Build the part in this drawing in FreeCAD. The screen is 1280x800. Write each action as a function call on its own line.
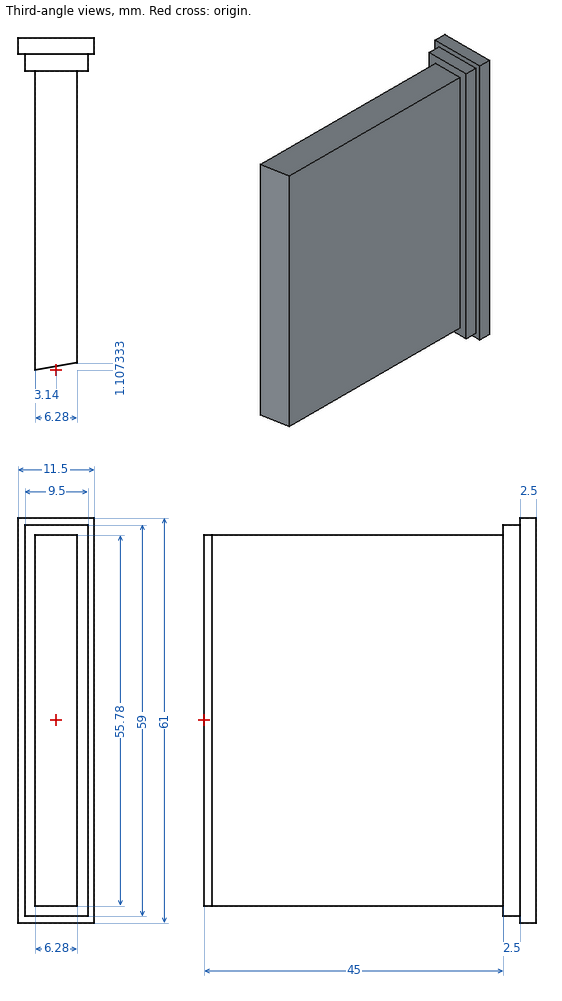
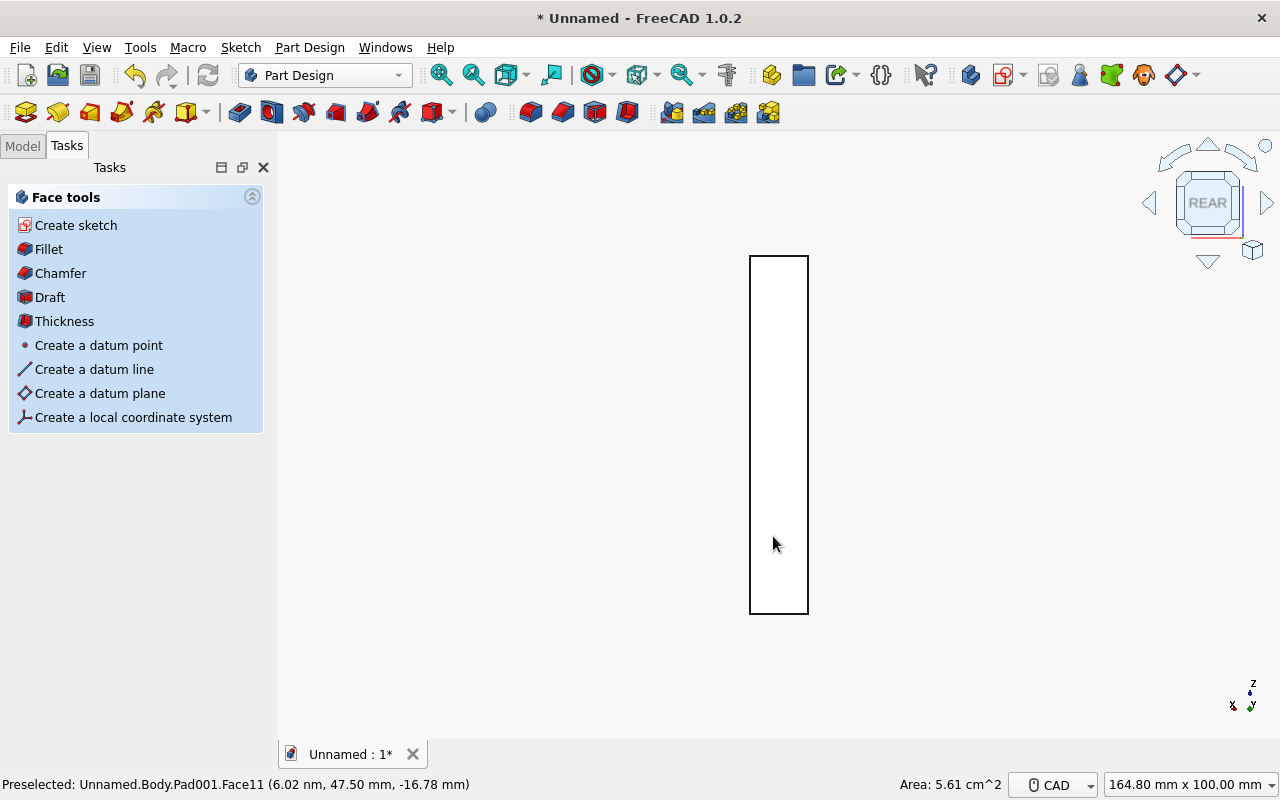
click(1004, 76)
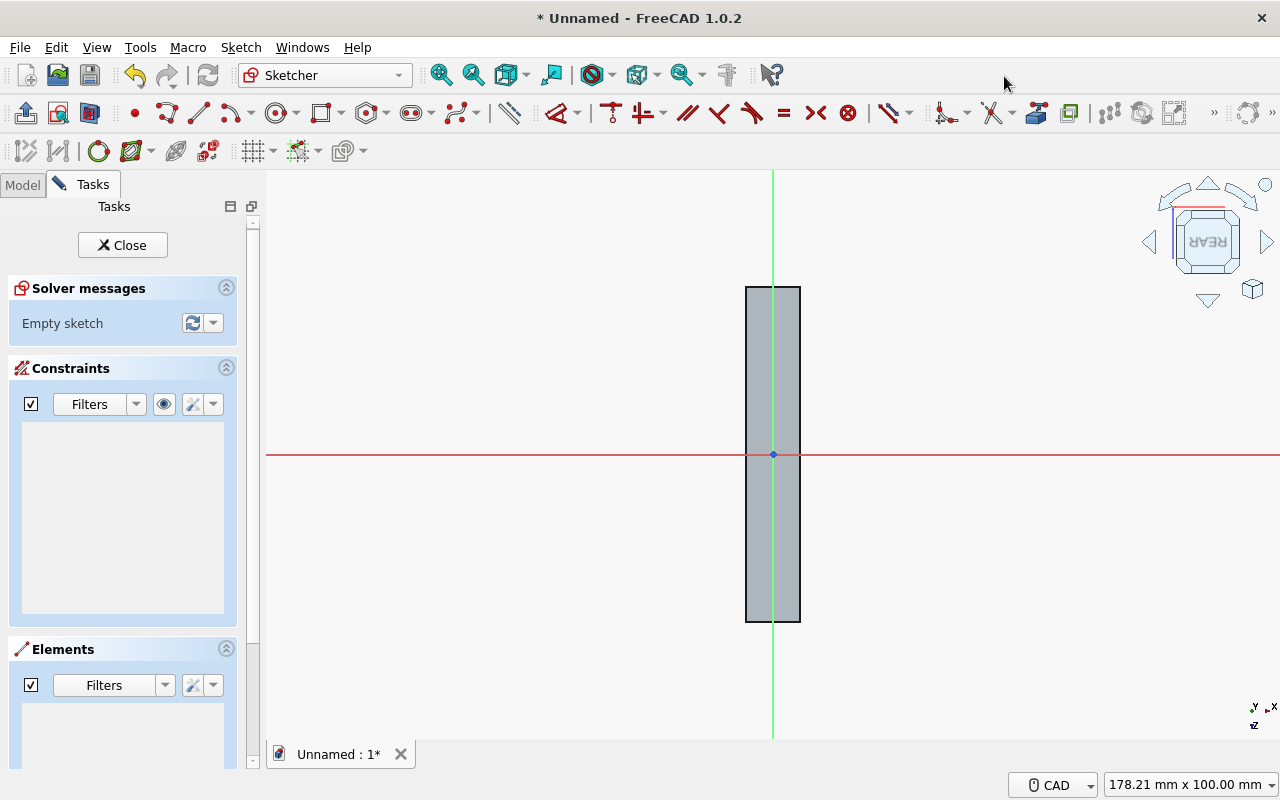
key(g)
key(v)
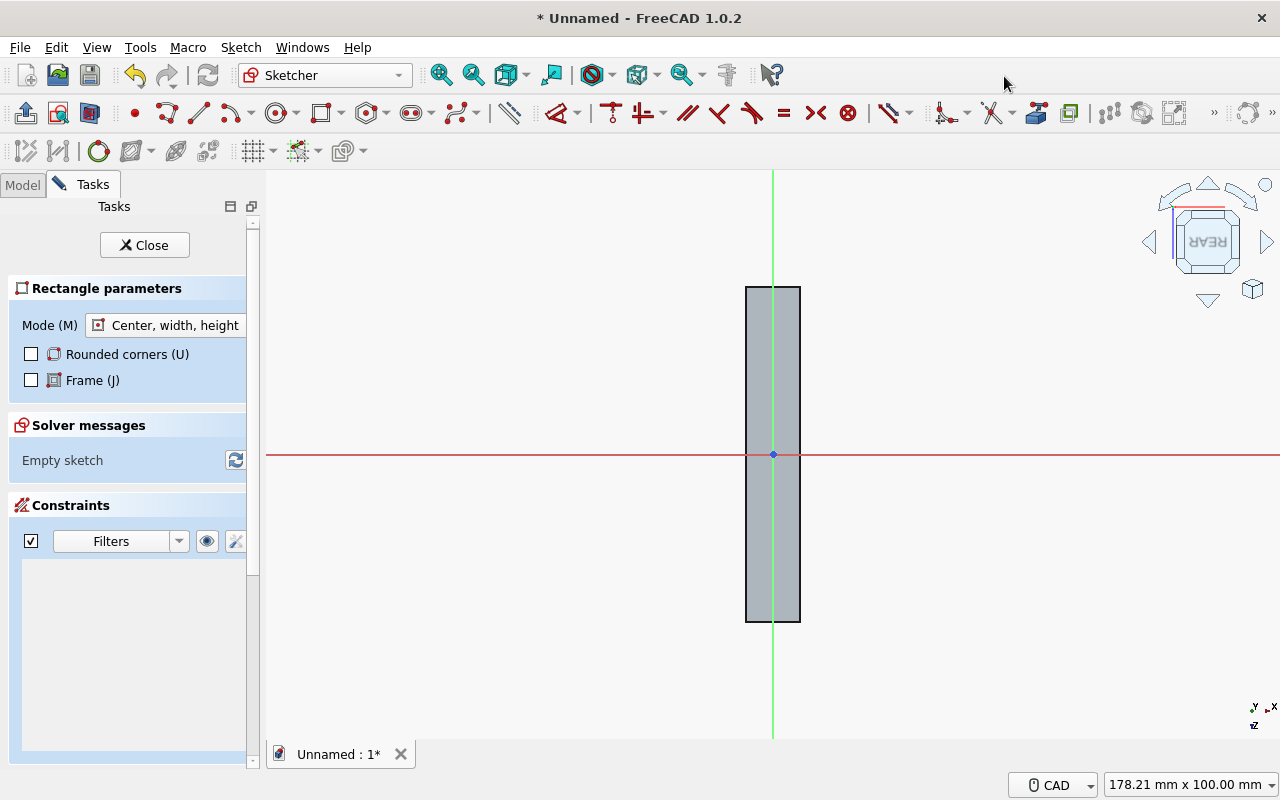
click(773, 454)
move(806, 281)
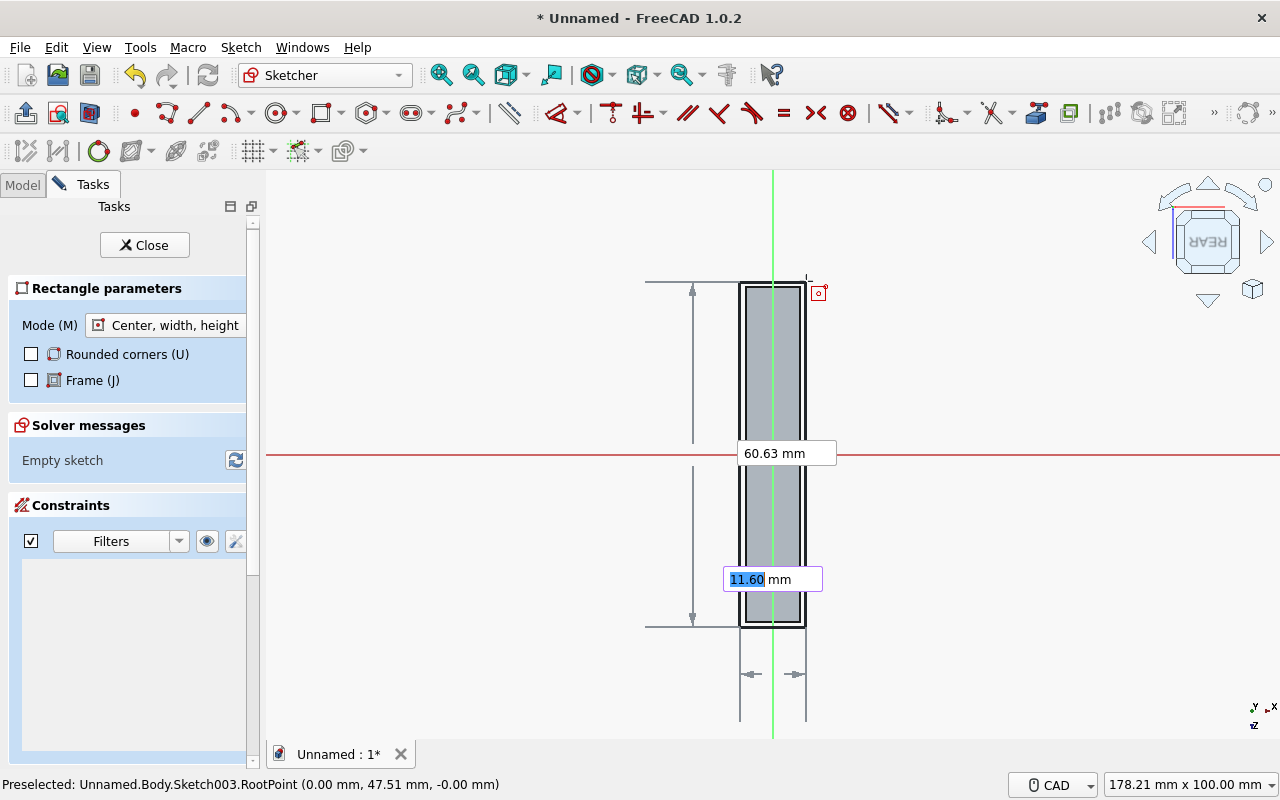
text(11.5)
key(Tab)
text(61)
key(Return)
key(Escape)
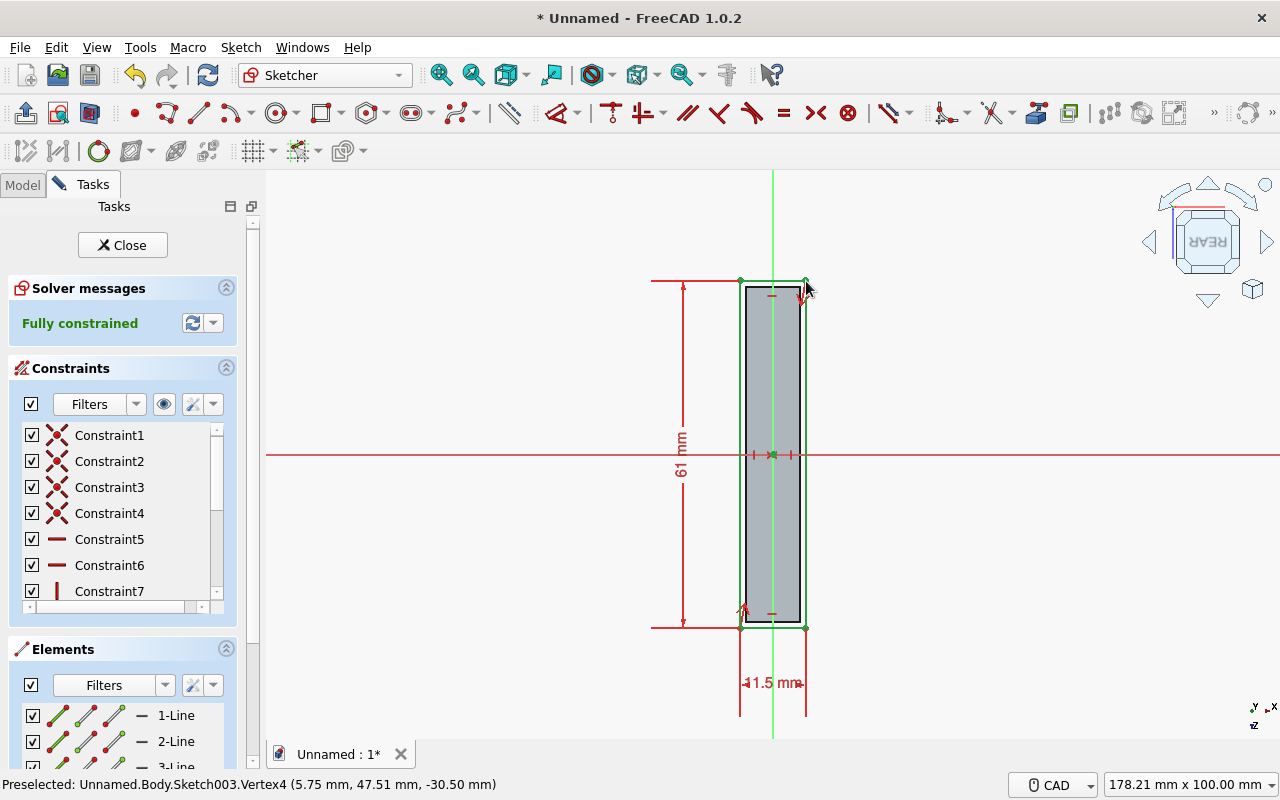
click(123, 245)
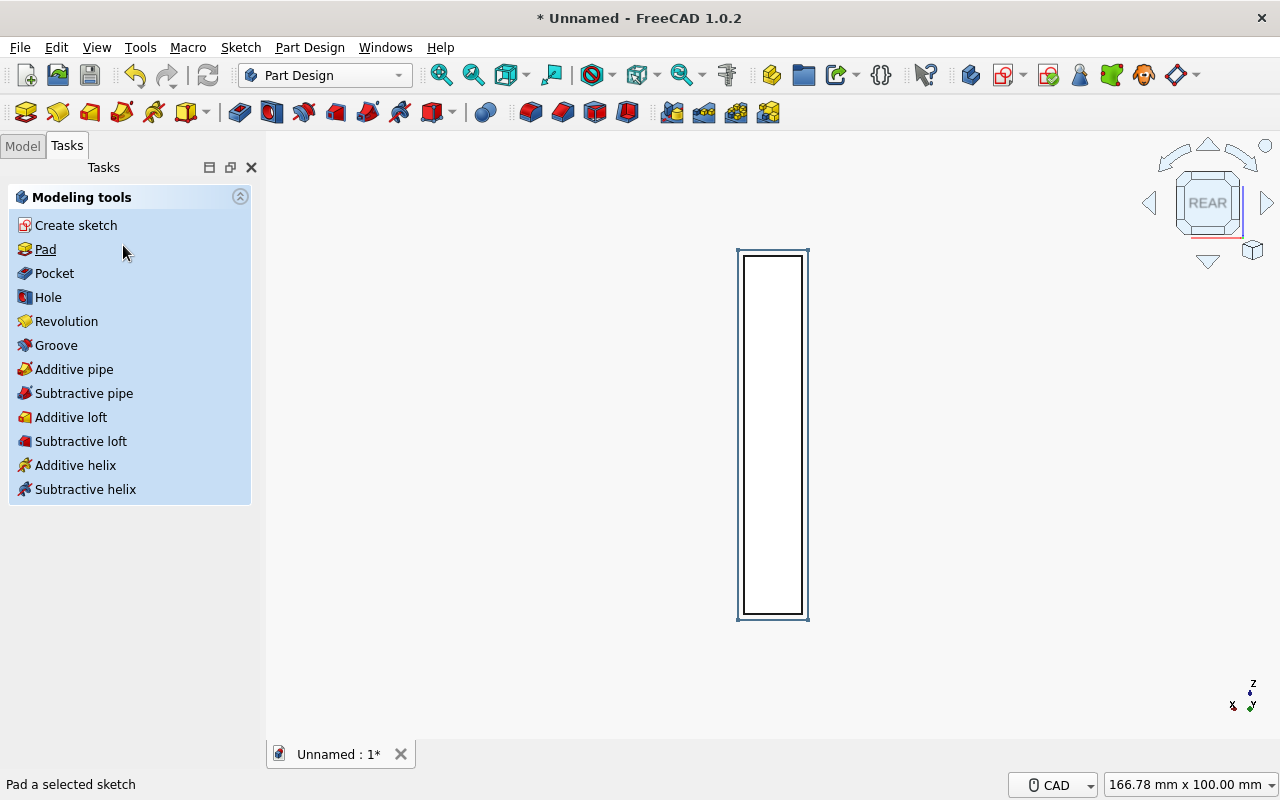
click(26, 112)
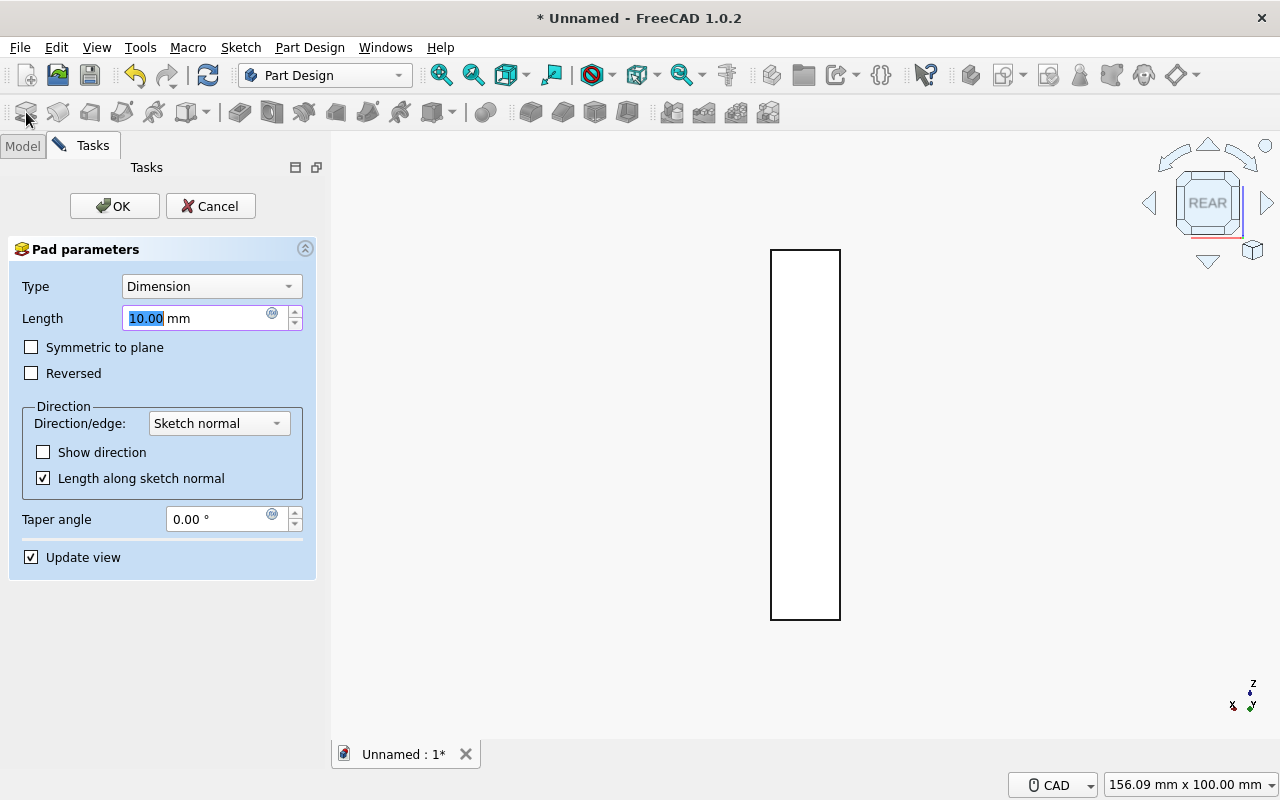
text(2.5)
key(Tab)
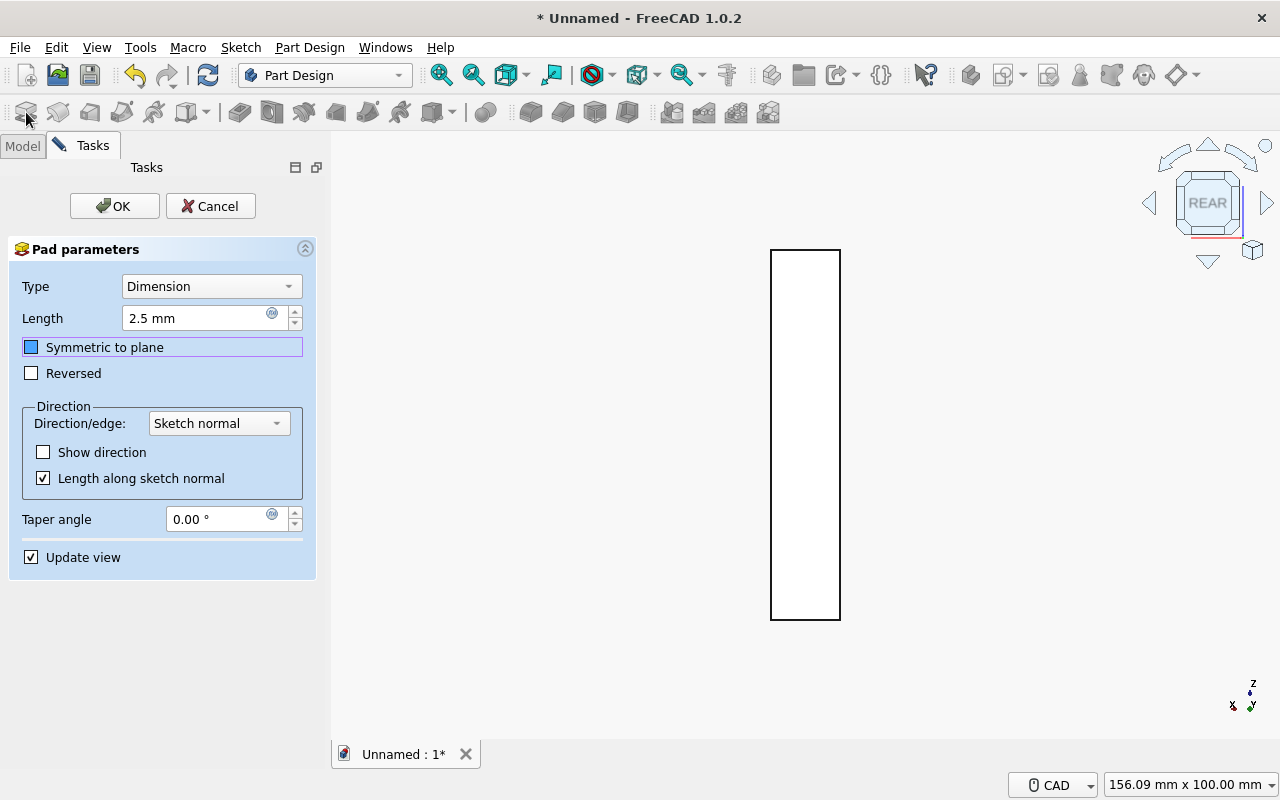
click(115, 206)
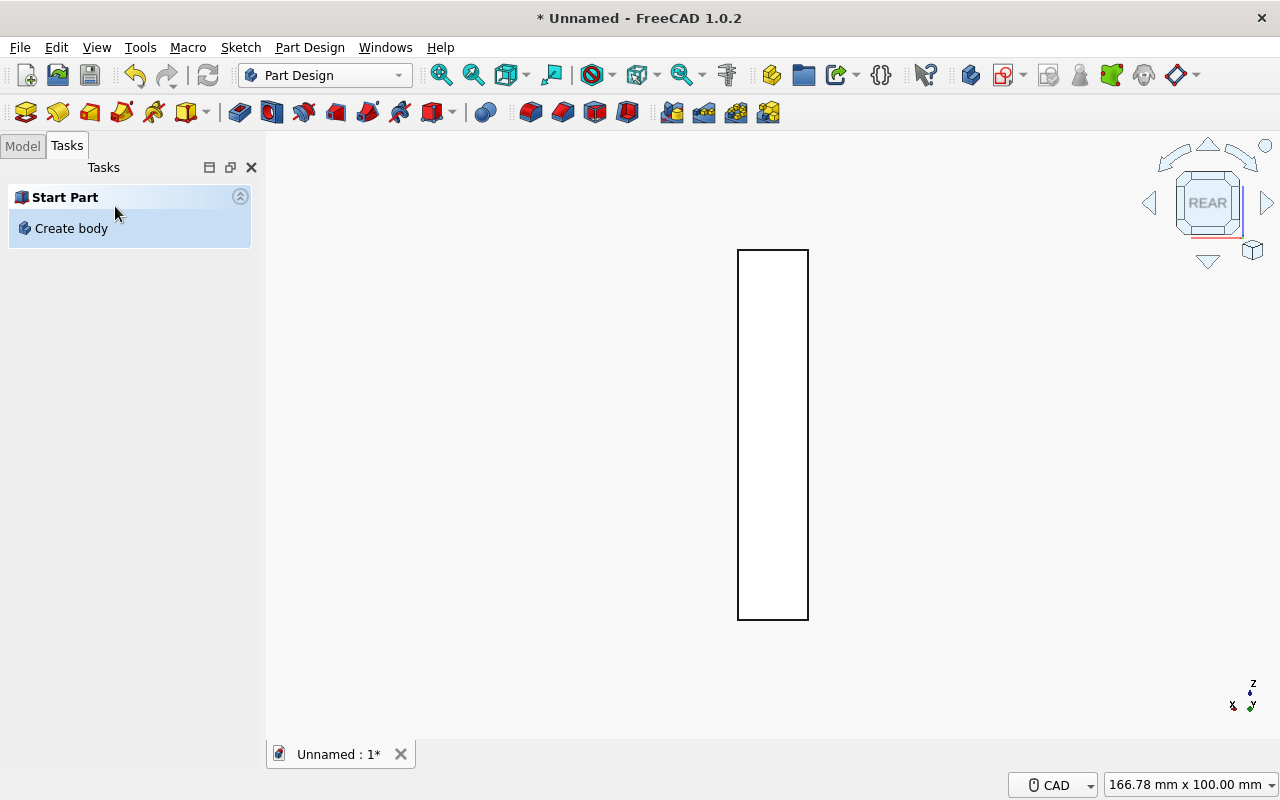
key(0)